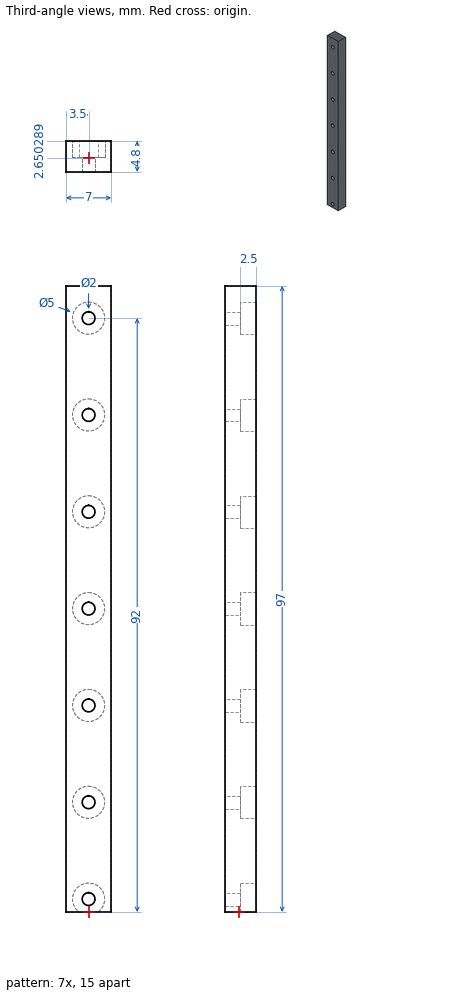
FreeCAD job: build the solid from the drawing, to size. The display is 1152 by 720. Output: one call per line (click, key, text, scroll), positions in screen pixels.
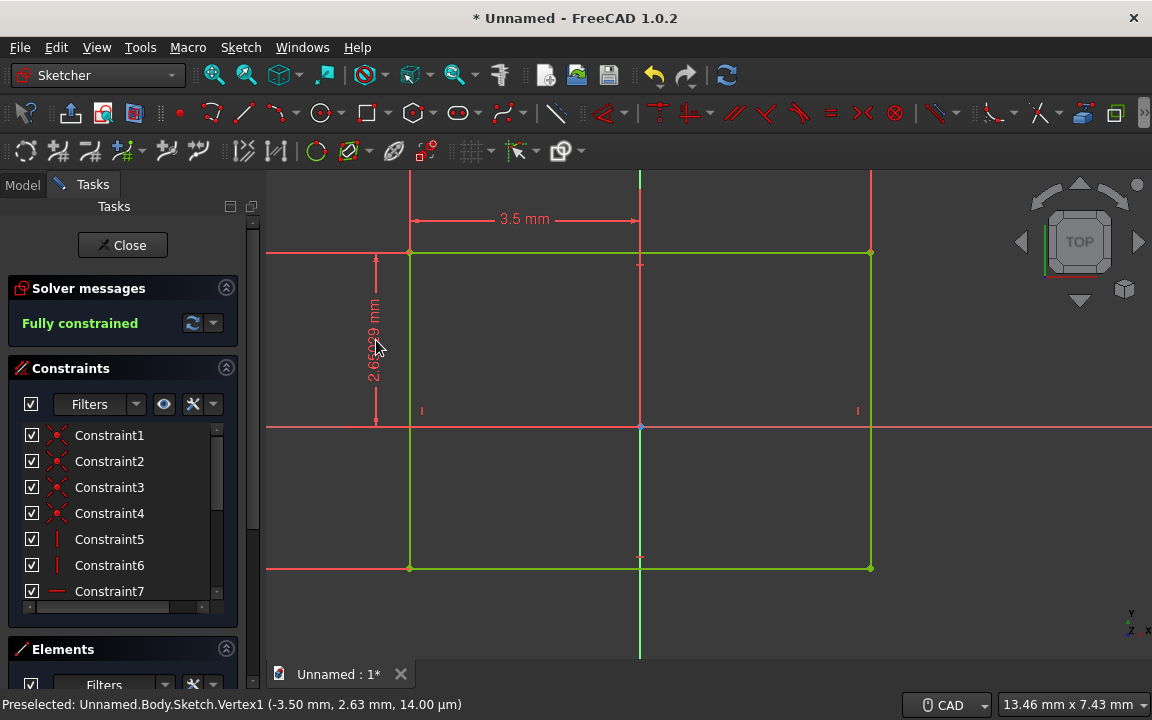
click(123, 245)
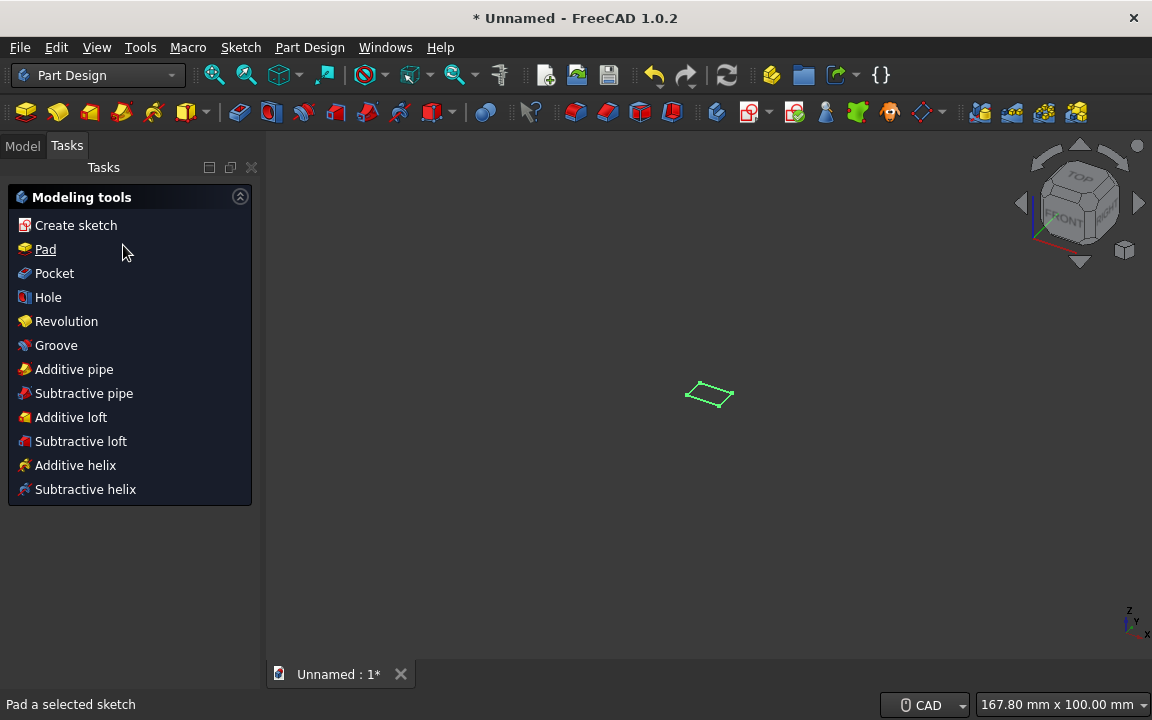
click(26, 112)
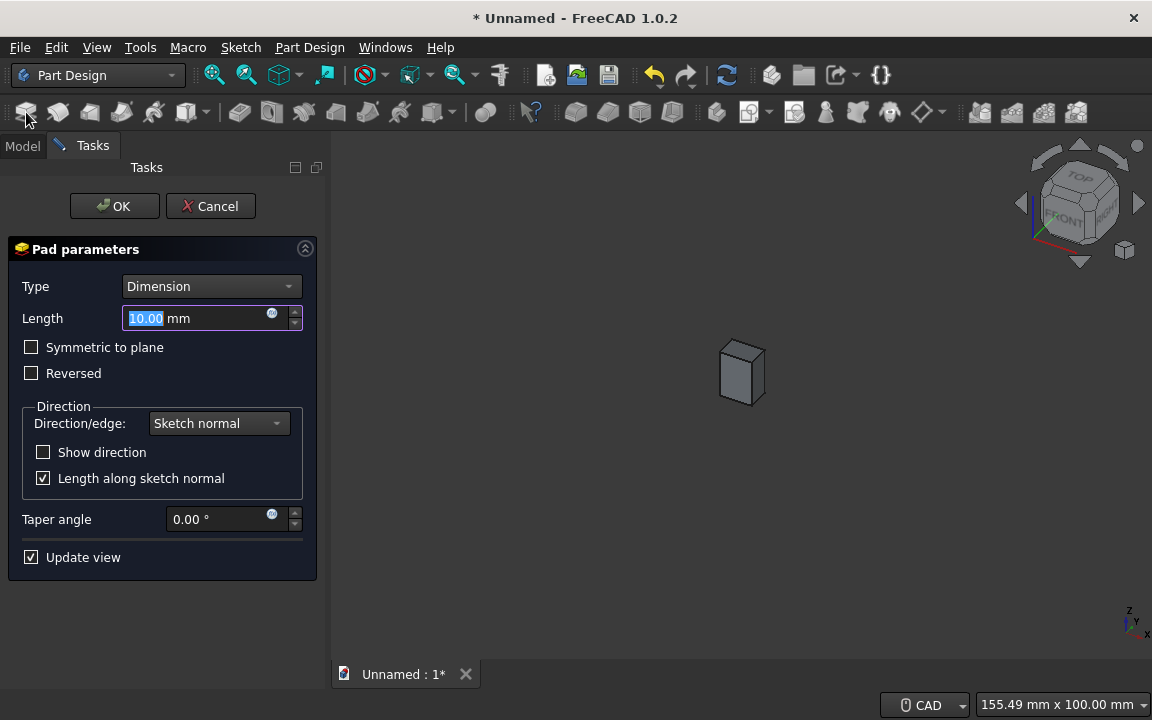
text(97)
key(Tab)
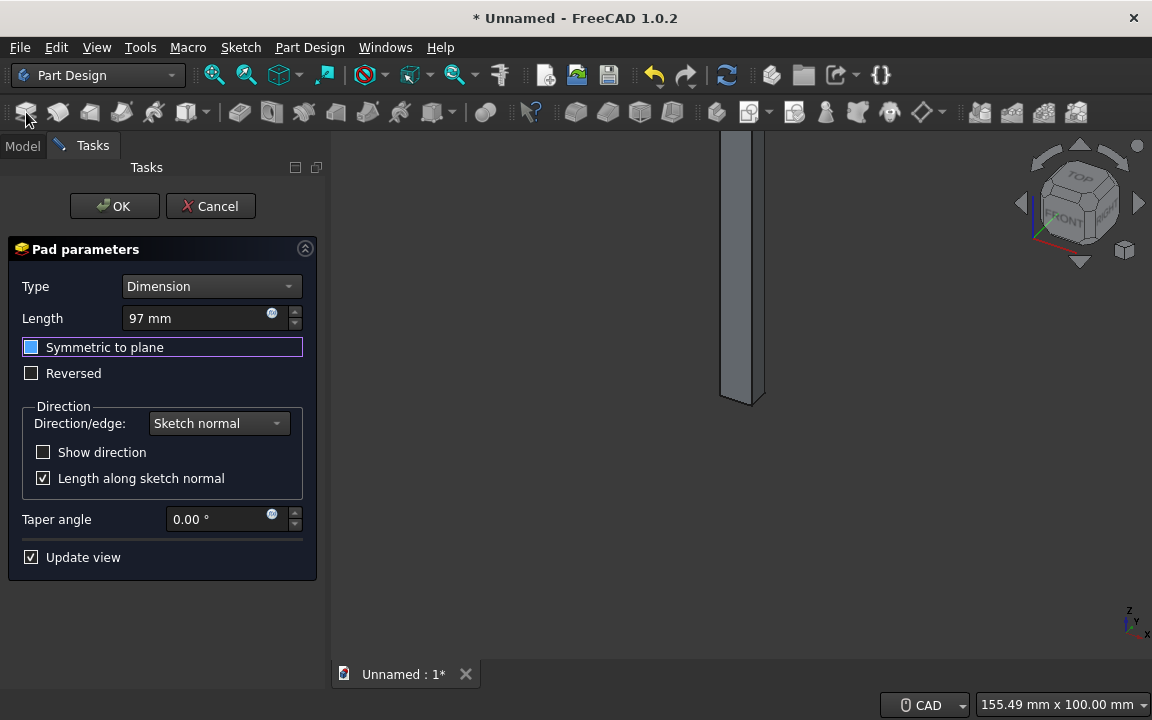
click(115, 206)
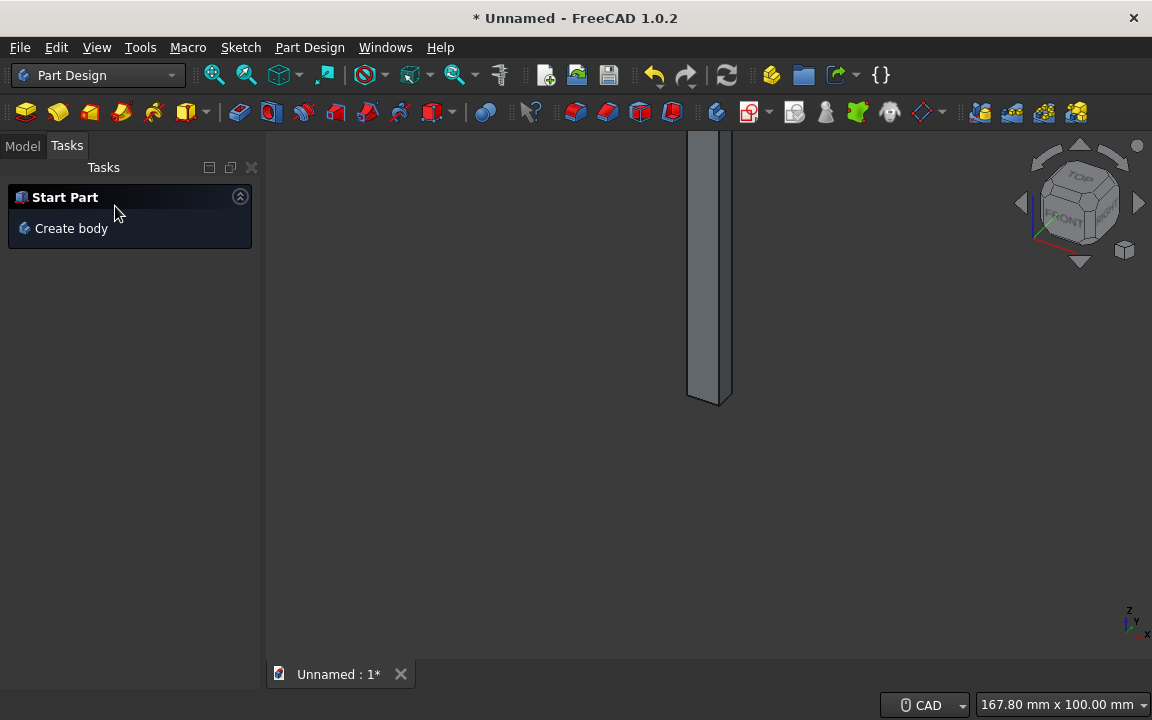
click(216, 76)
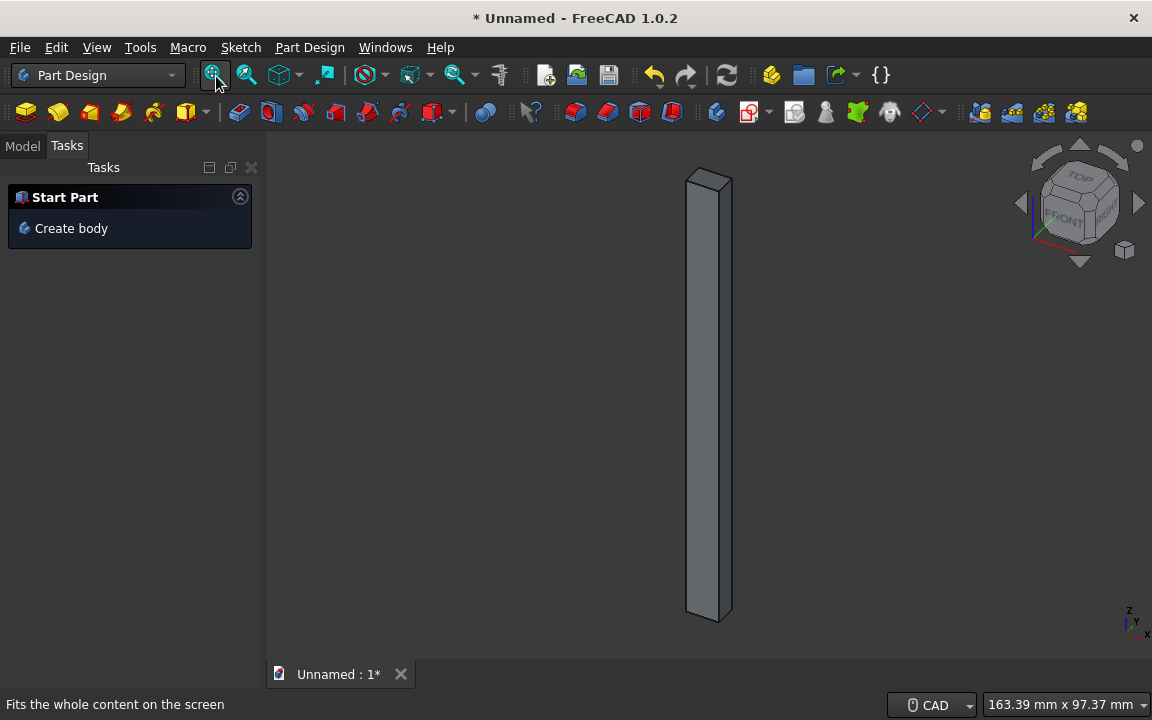
key(4)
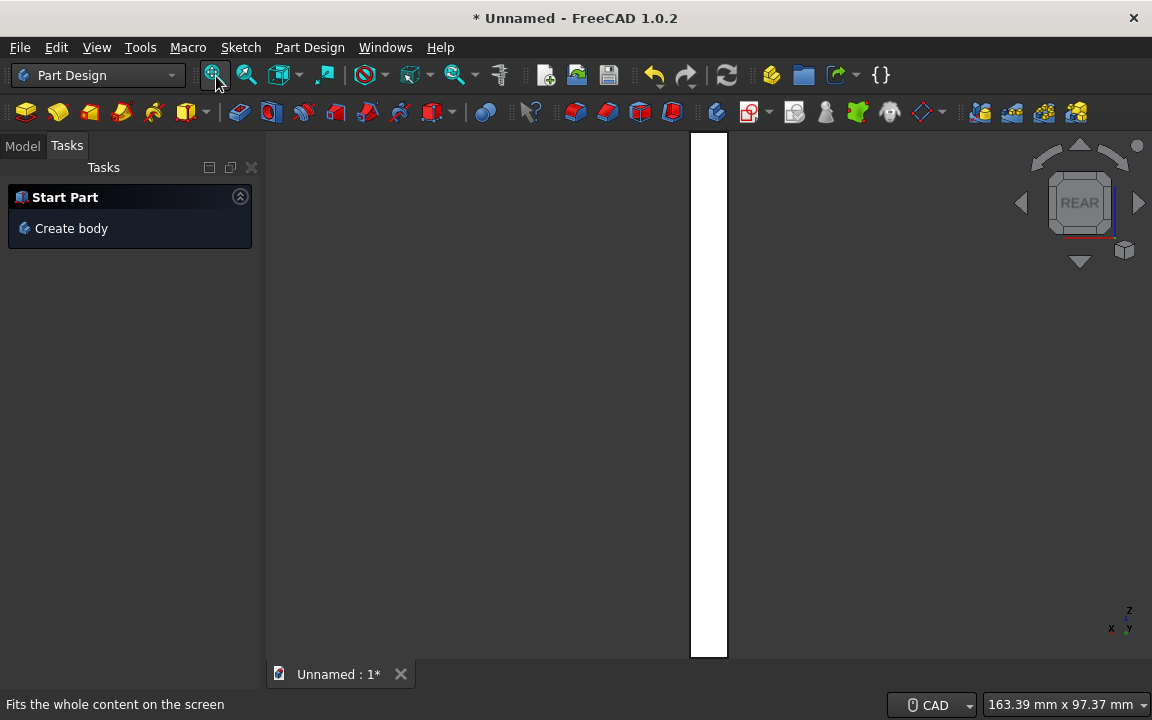
click(709, 169)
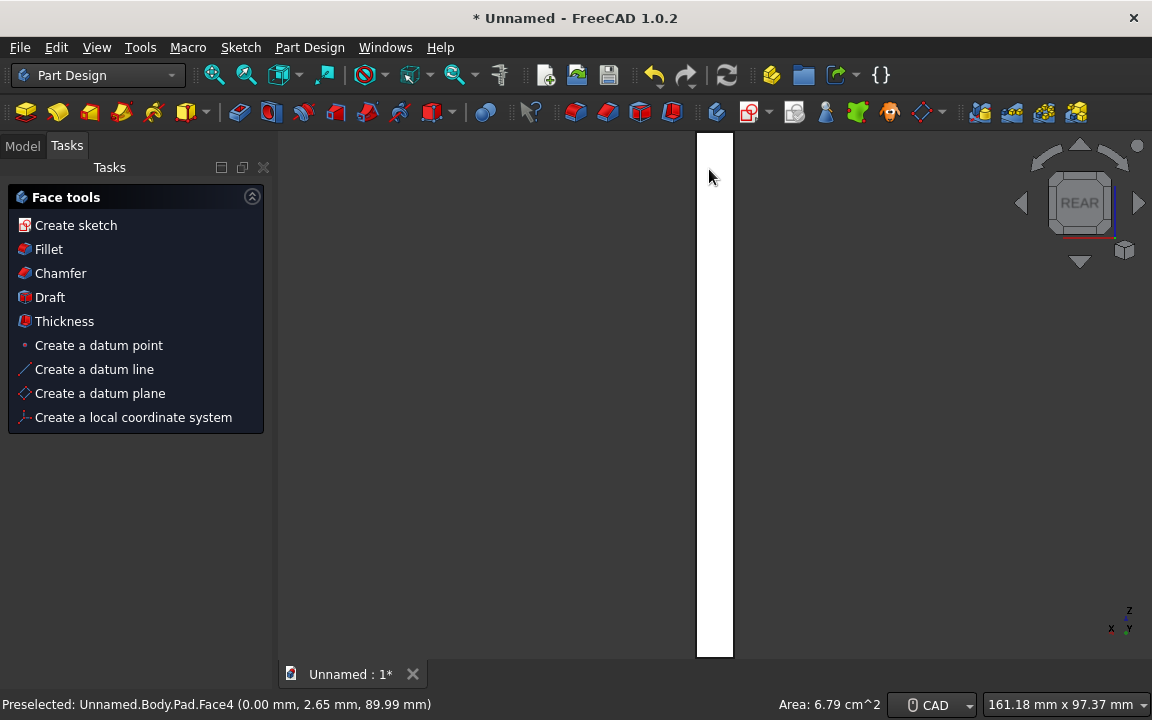
click(750, 112)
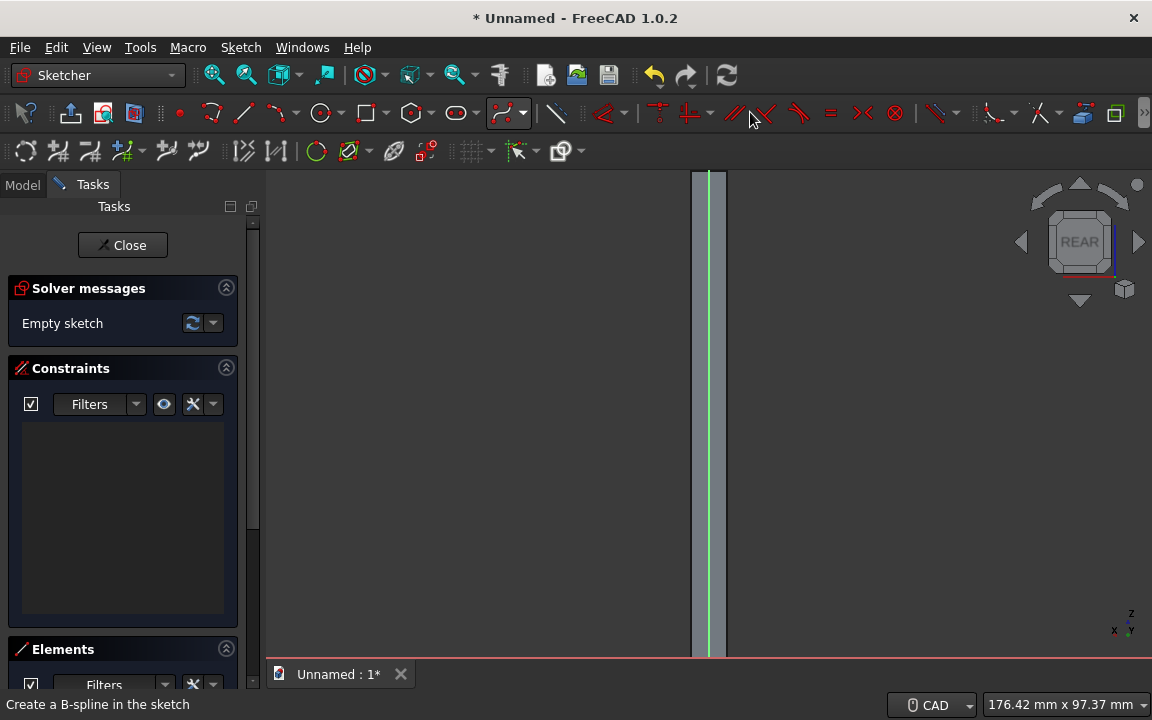
scroll(640, 414, down, 5)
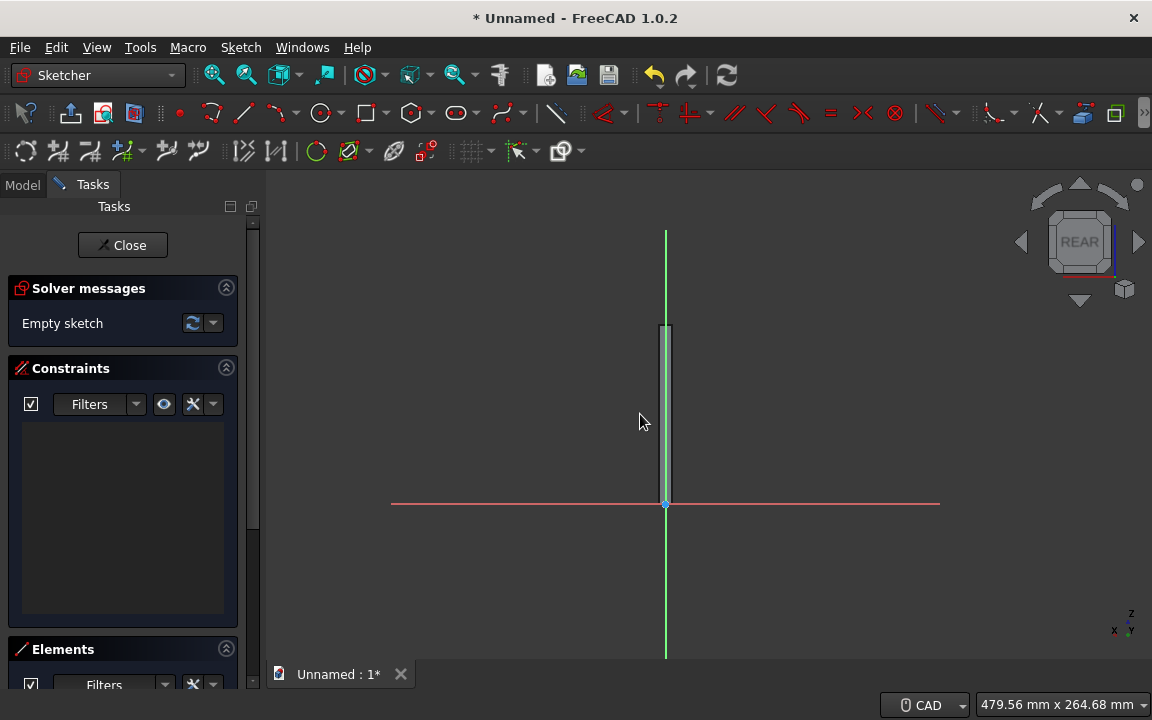
scroll(667, 330, up, 15)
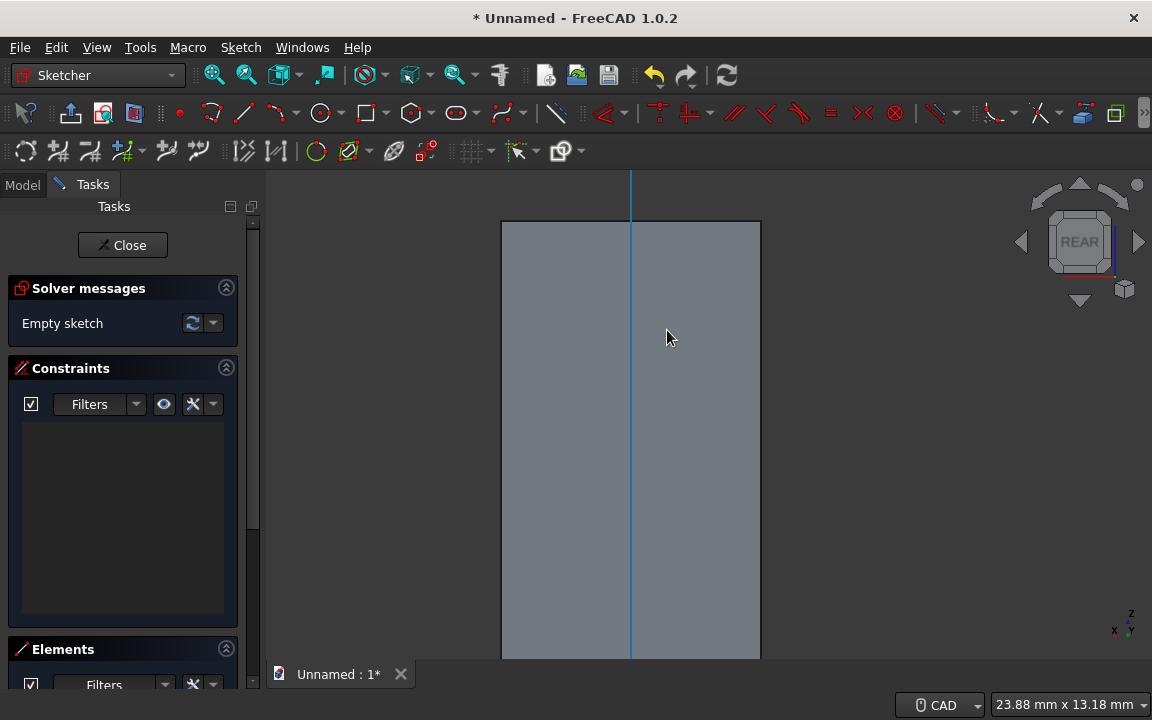
scroll(628, 404, up, 7)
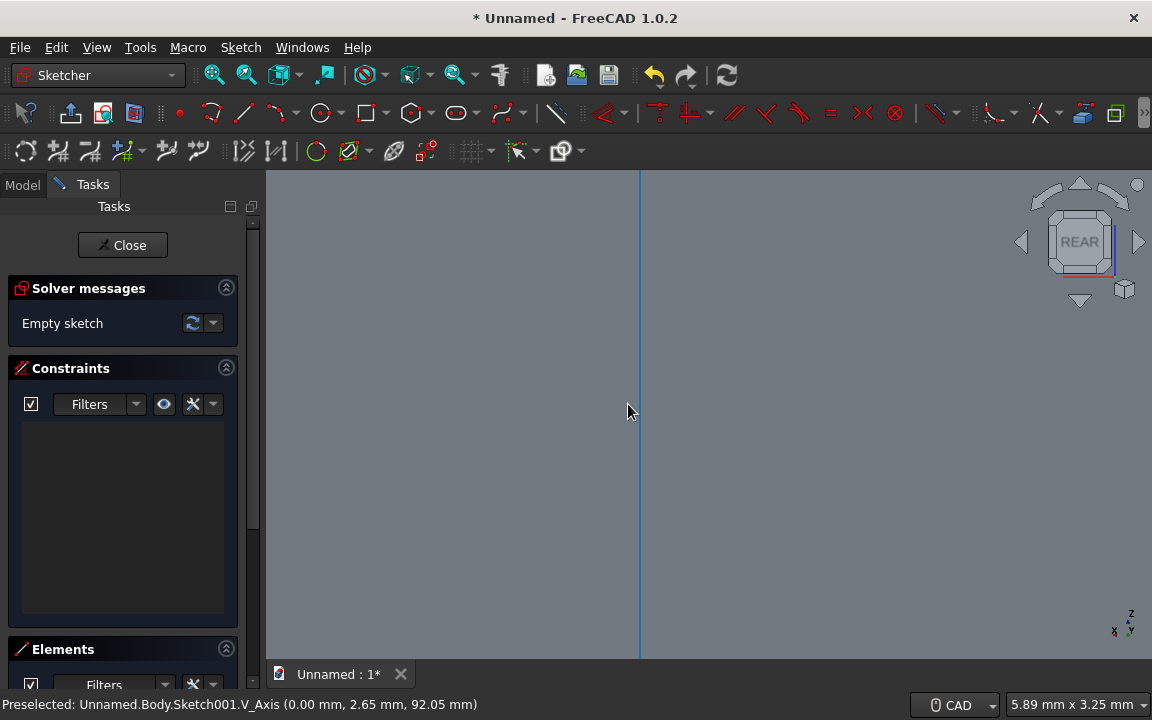
key(g)
key(c)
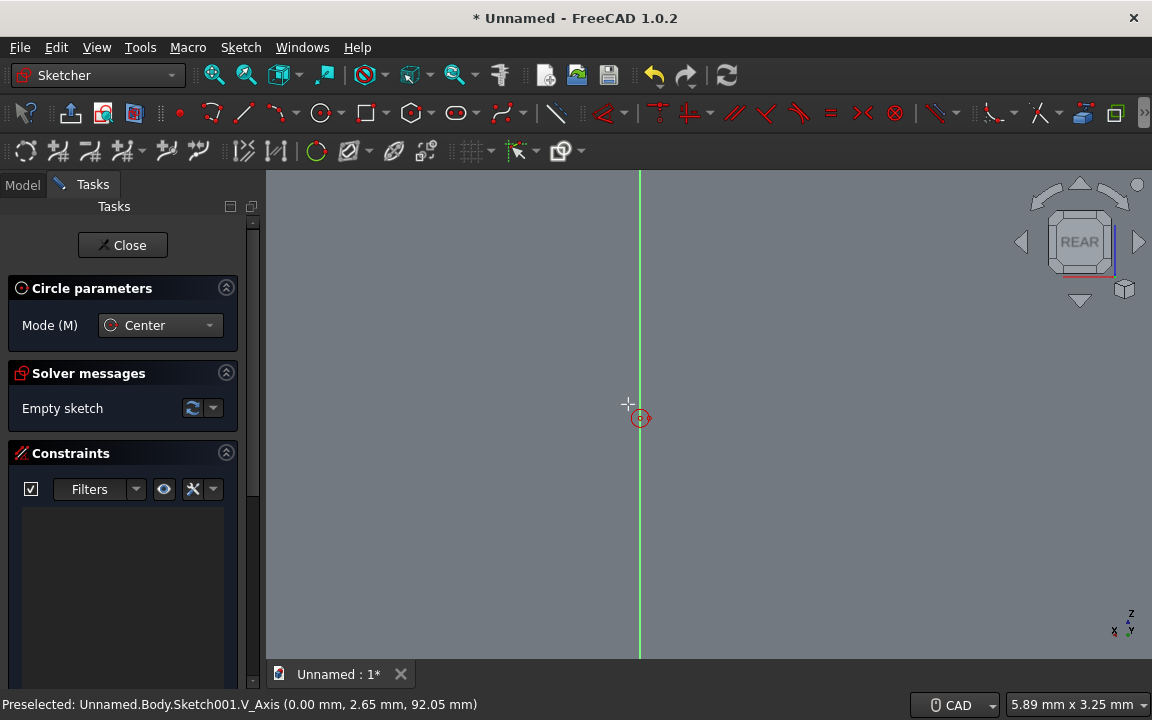
click(640, 414)
move(746, 307)